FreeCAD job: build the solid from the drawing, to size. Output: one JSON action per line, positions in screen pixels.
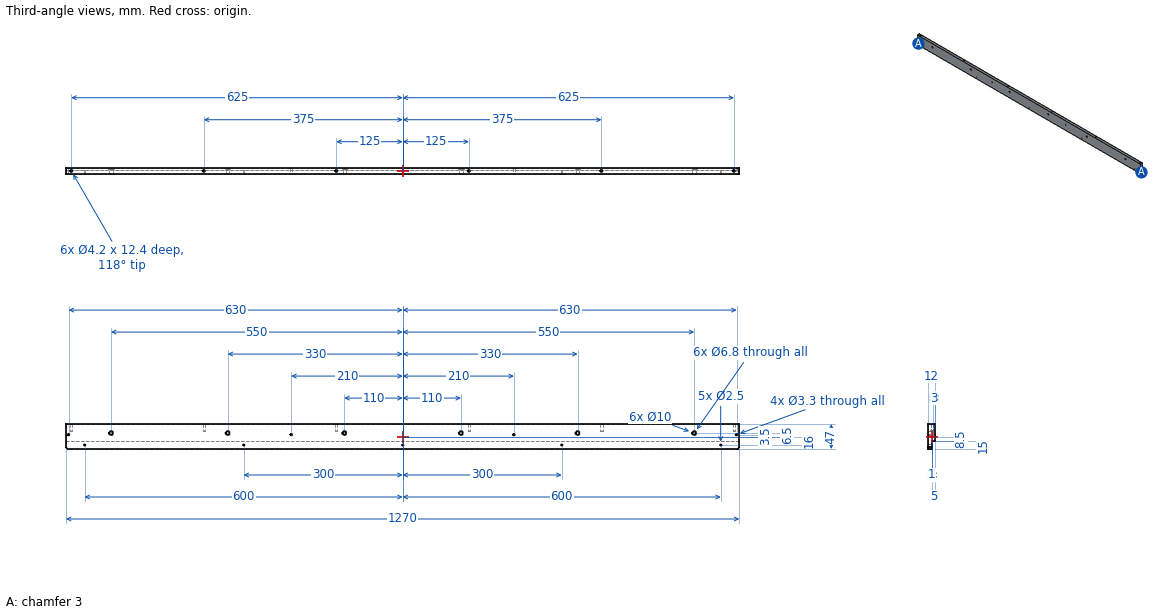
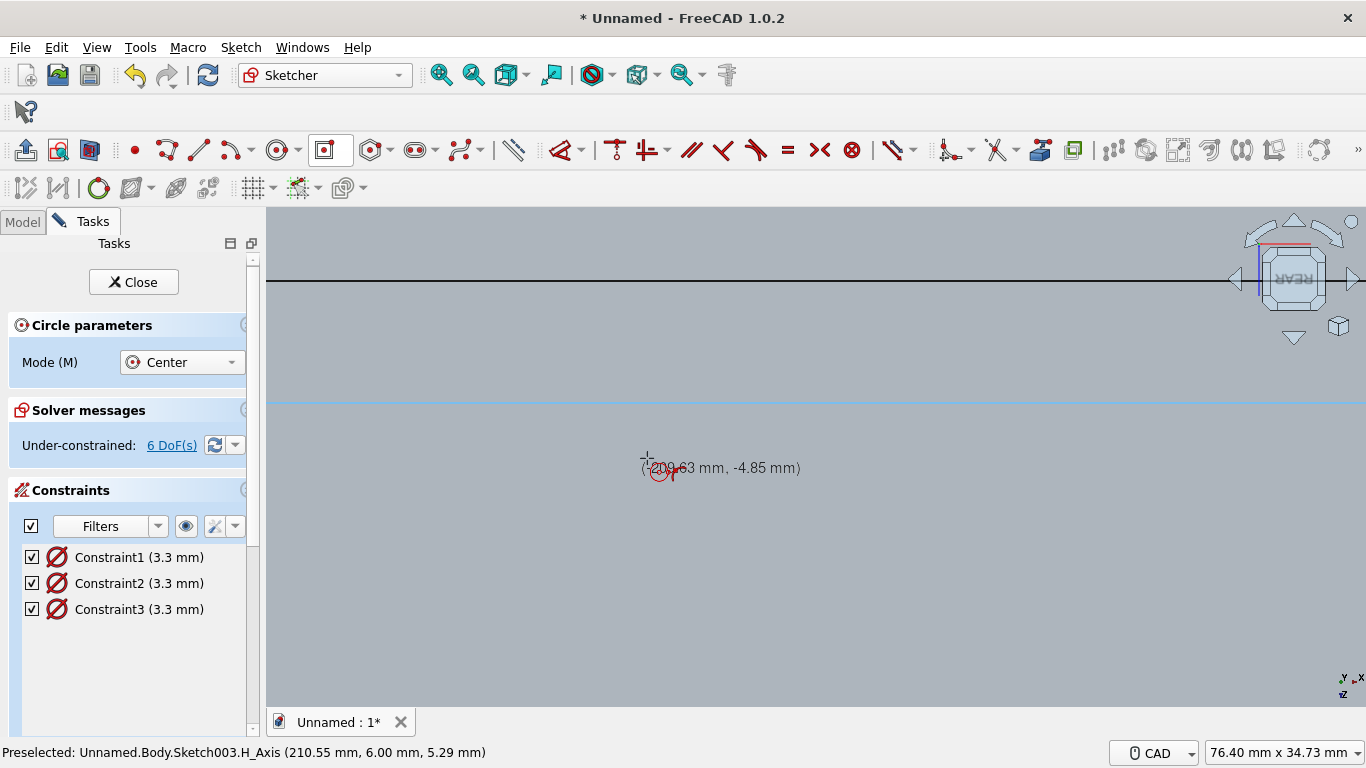
{"action": "scroll", "coordinate": [624, 458], "scroll_direction": "down", "scroll_amount": 16}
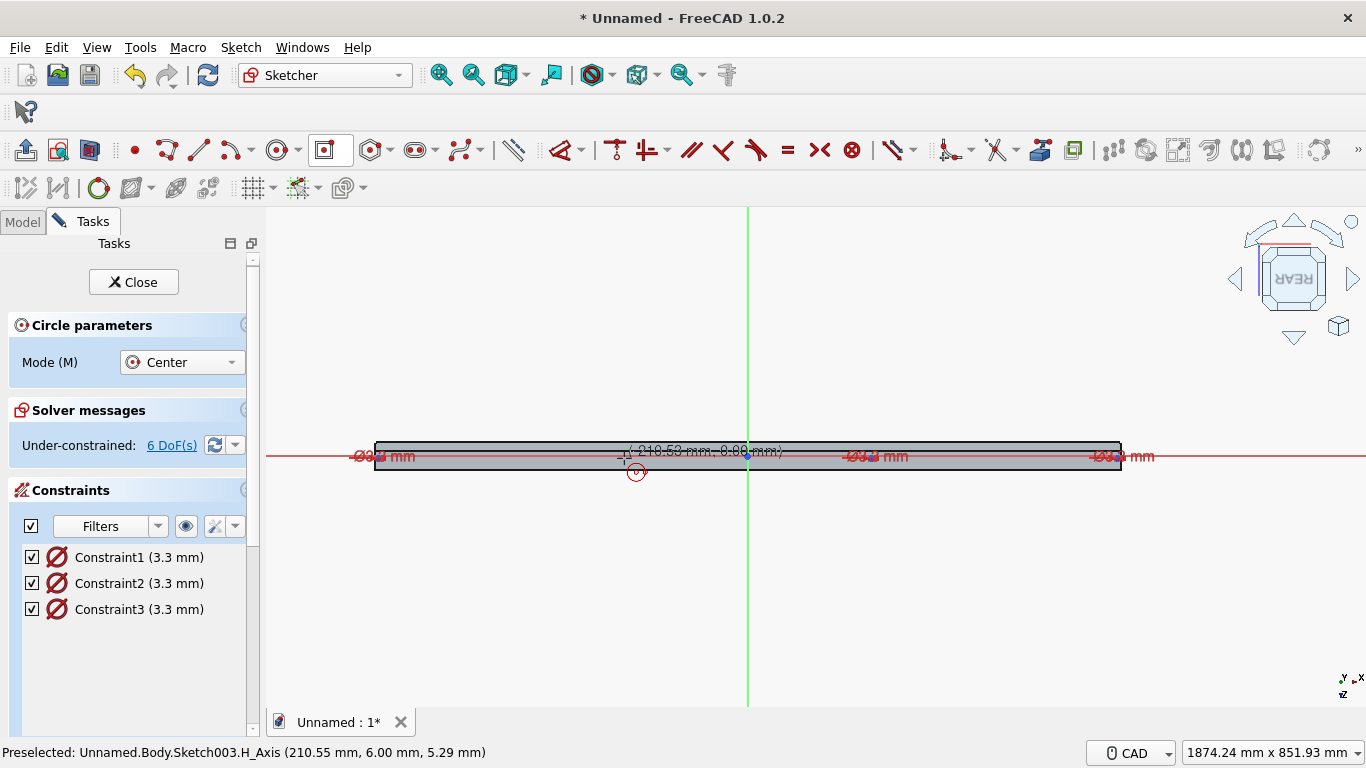
{"action": "scroll", "coordinate": [625, 458], "scroll_direction": "up", "scroll_amount": 11}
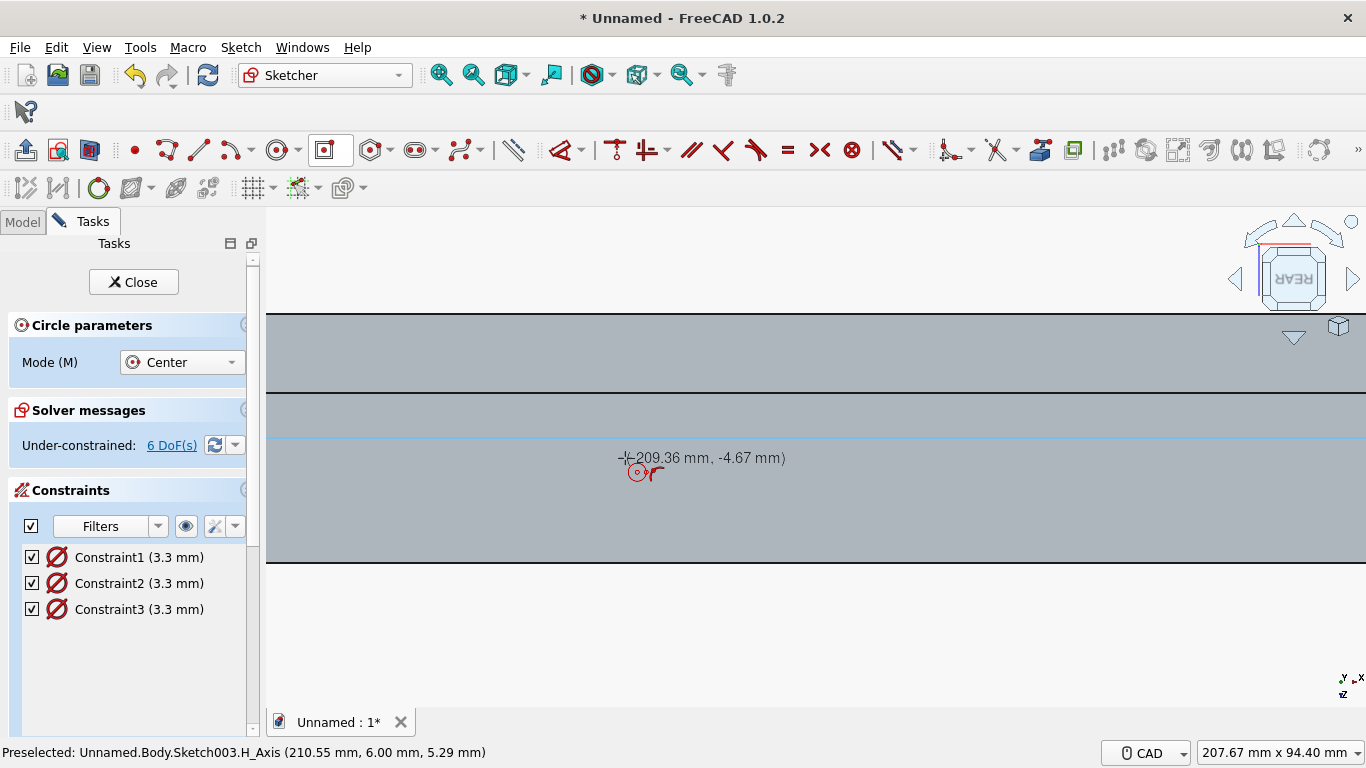
{"action": "left_click", "coordinate": [619, 457]}
{"action": "mouse_move", "coordinate": [625, 463]}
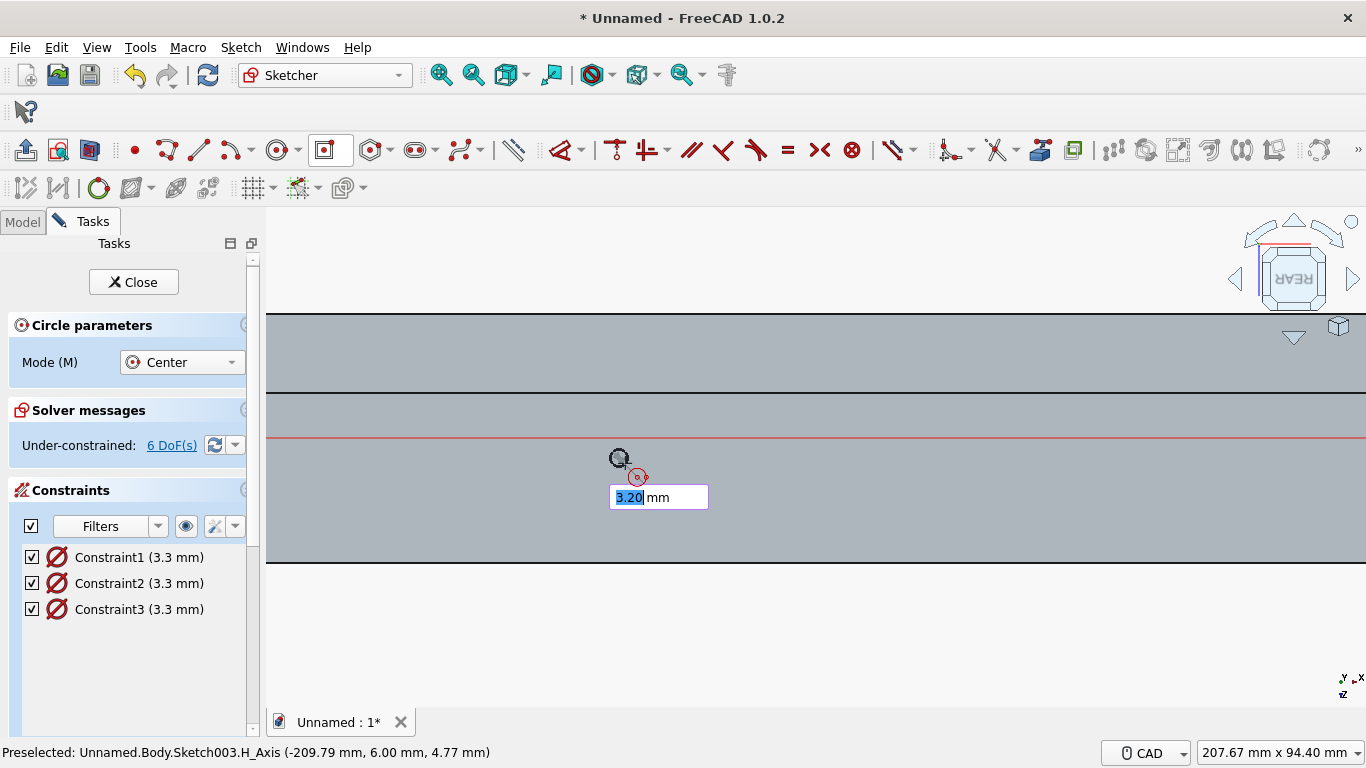
{"action": "type", "text": "3.3"}
{"action": "key", "text": "Return"}
{"action": "key", "text": "Escape"}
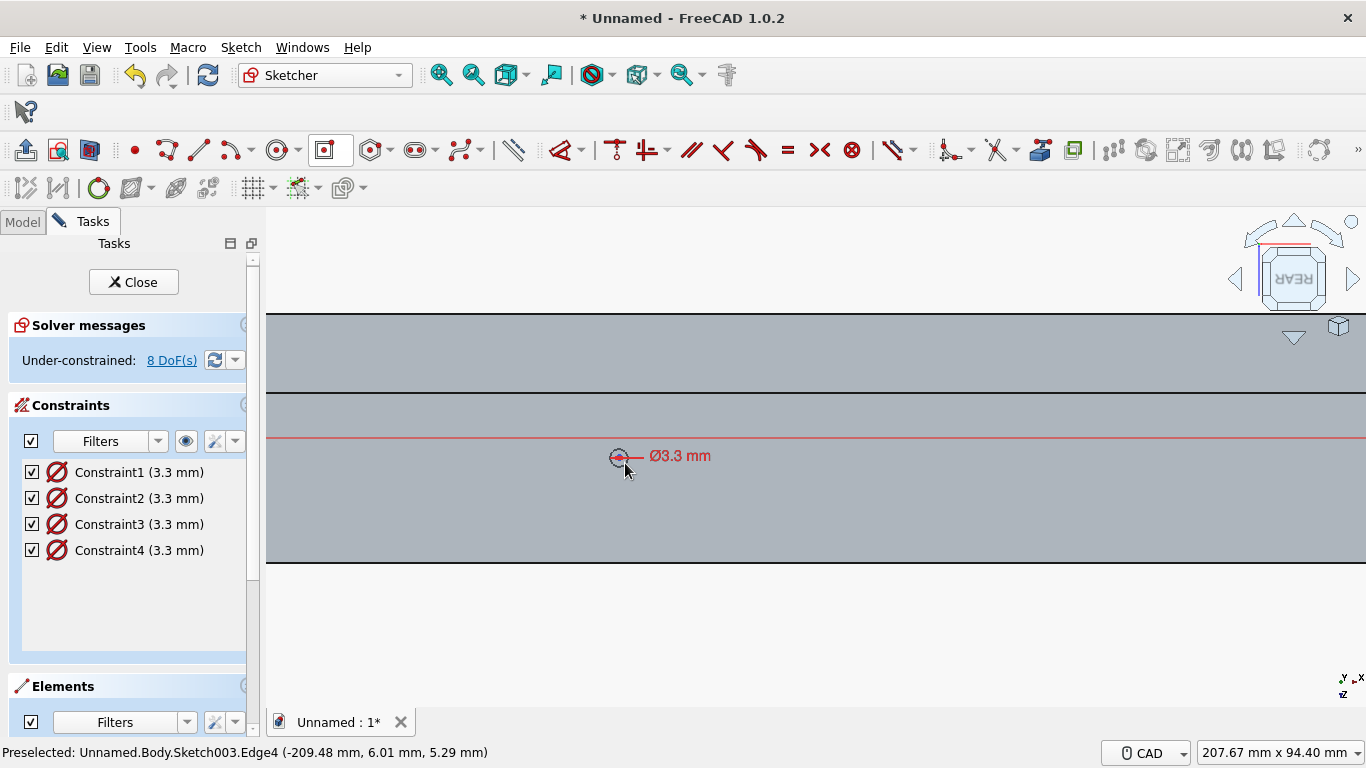
{"action": "scroll", "coordinate": [649, 458], "scroll_direction": "down", "scroll_amount": 12}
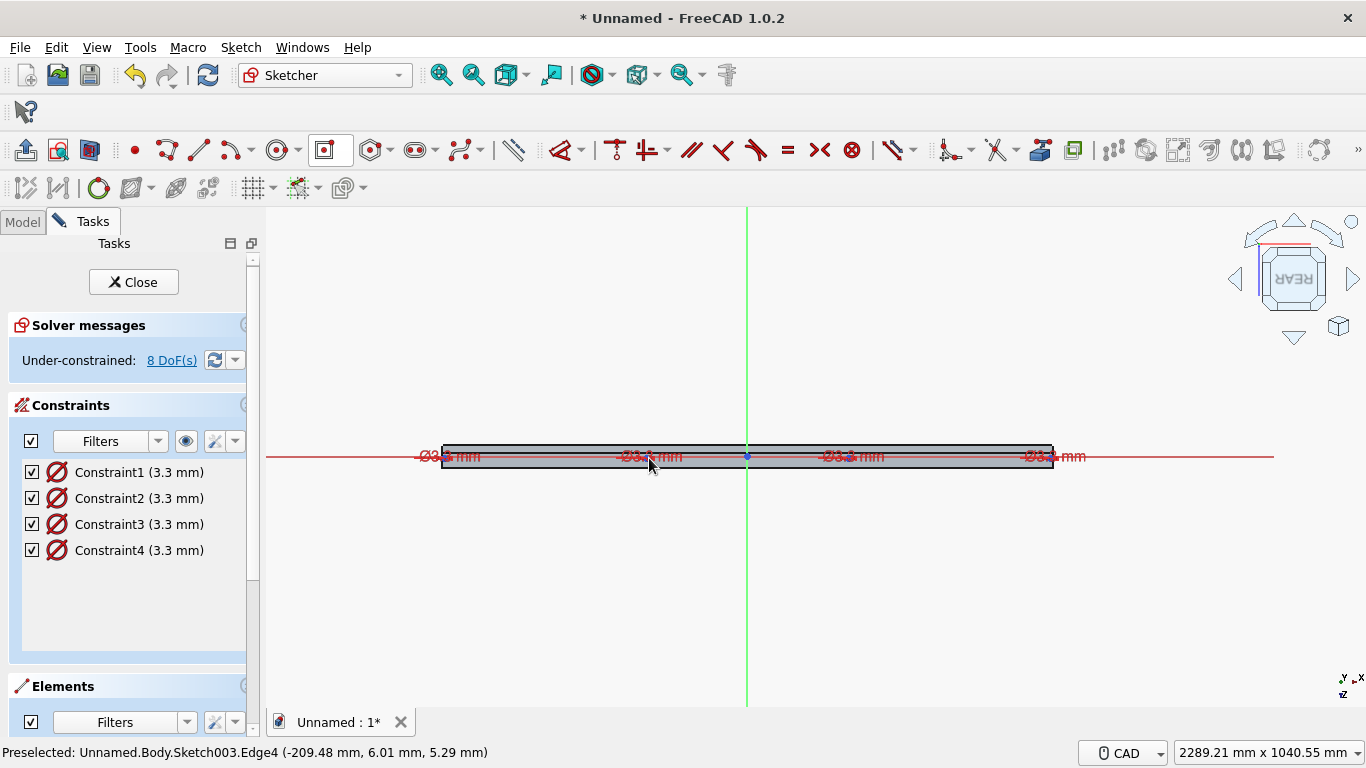
{"action": "left_click", "coordinate": [1050, 458]}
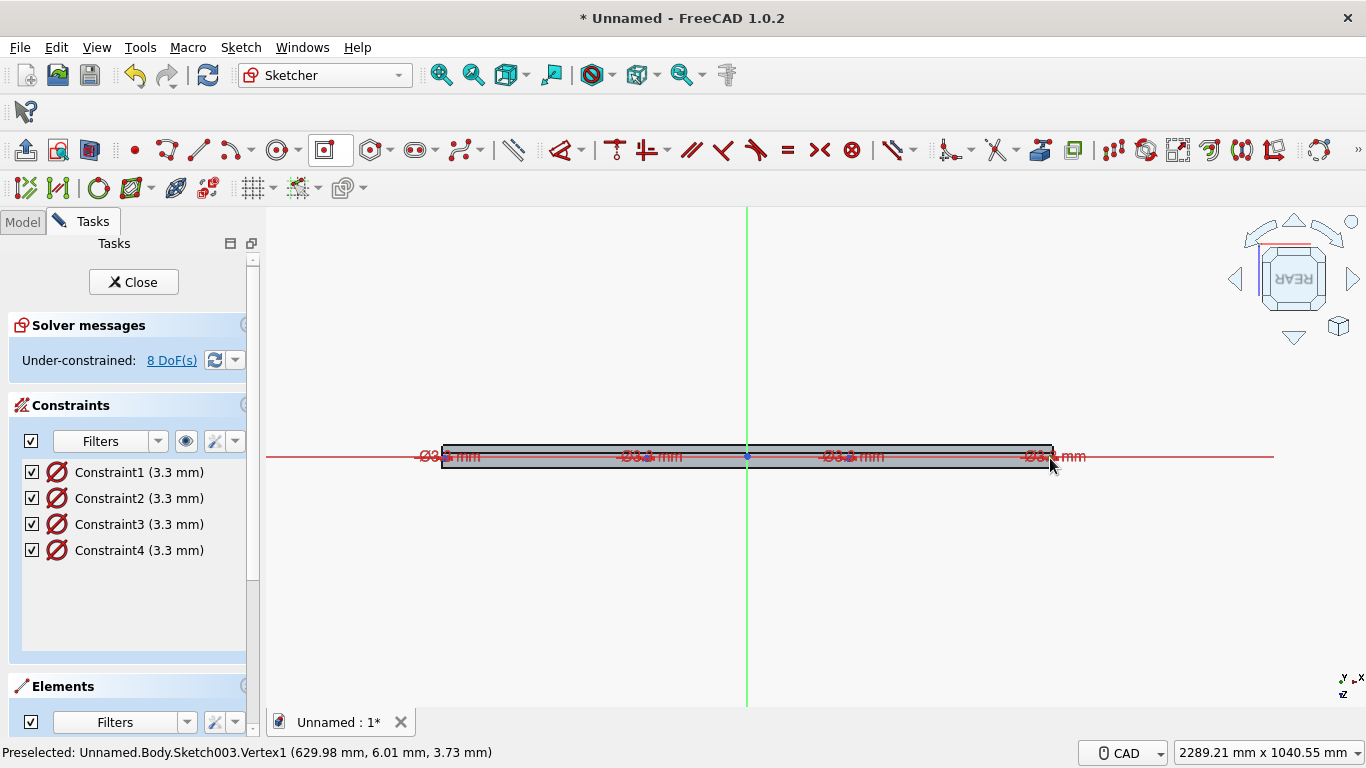
{"action": "left_click", "coordinate": [445, 458]}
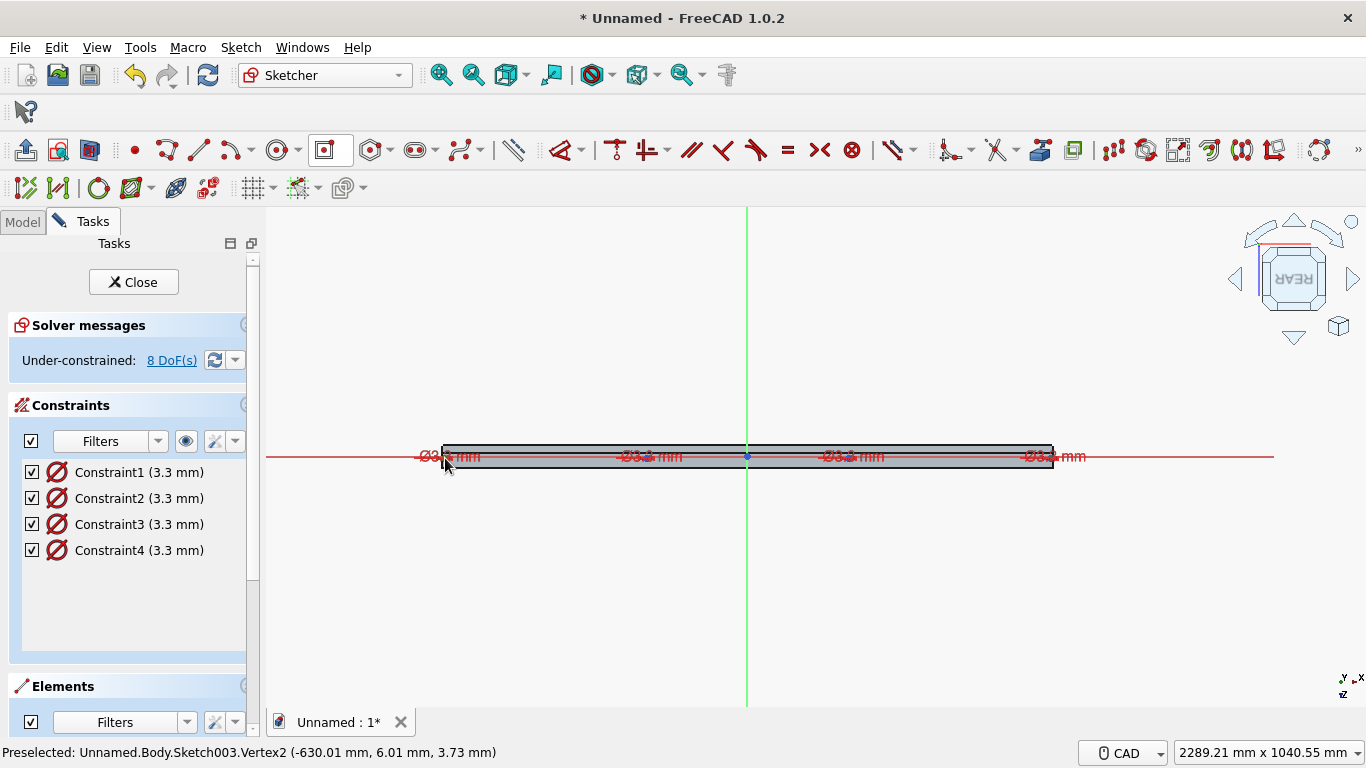
{"action": "left_click", "coordinate": [670, 150]}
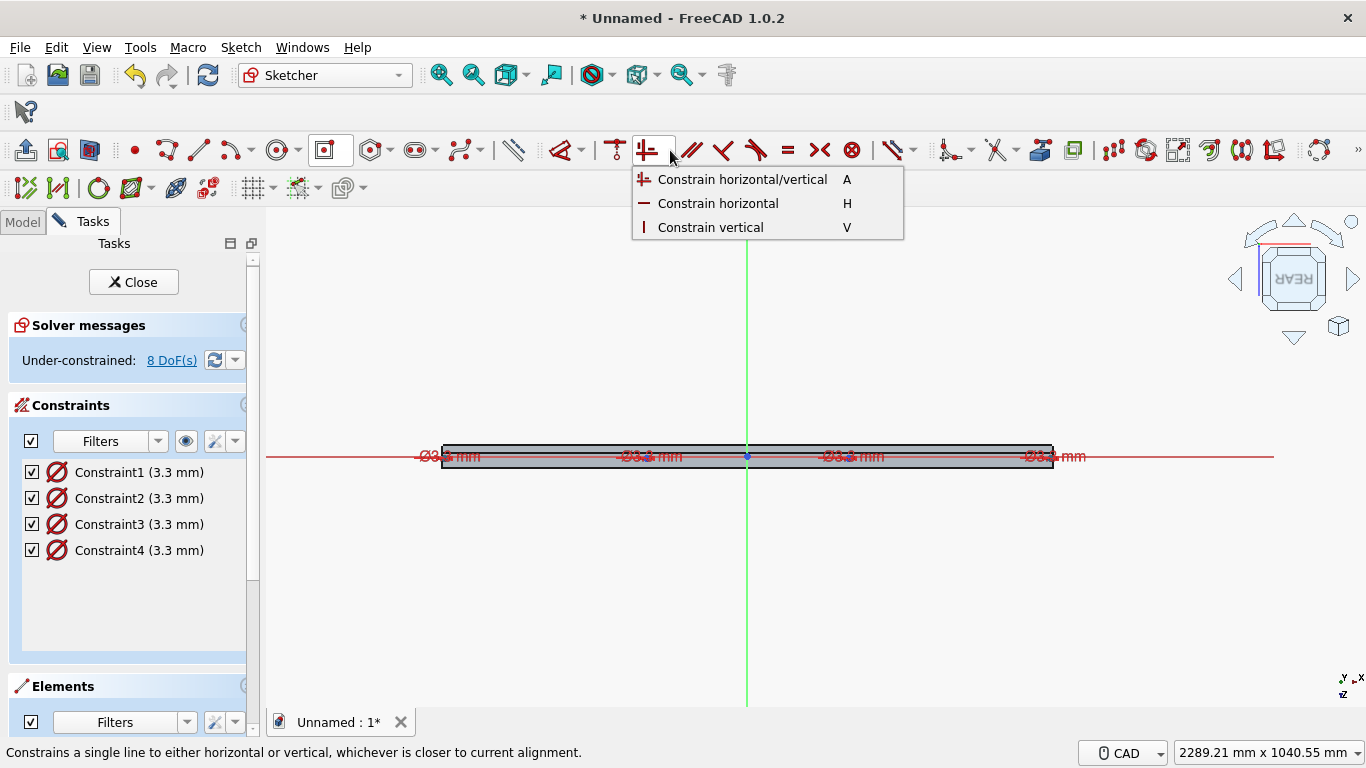
{"action": "left_click", "coordinate": [768, 203]}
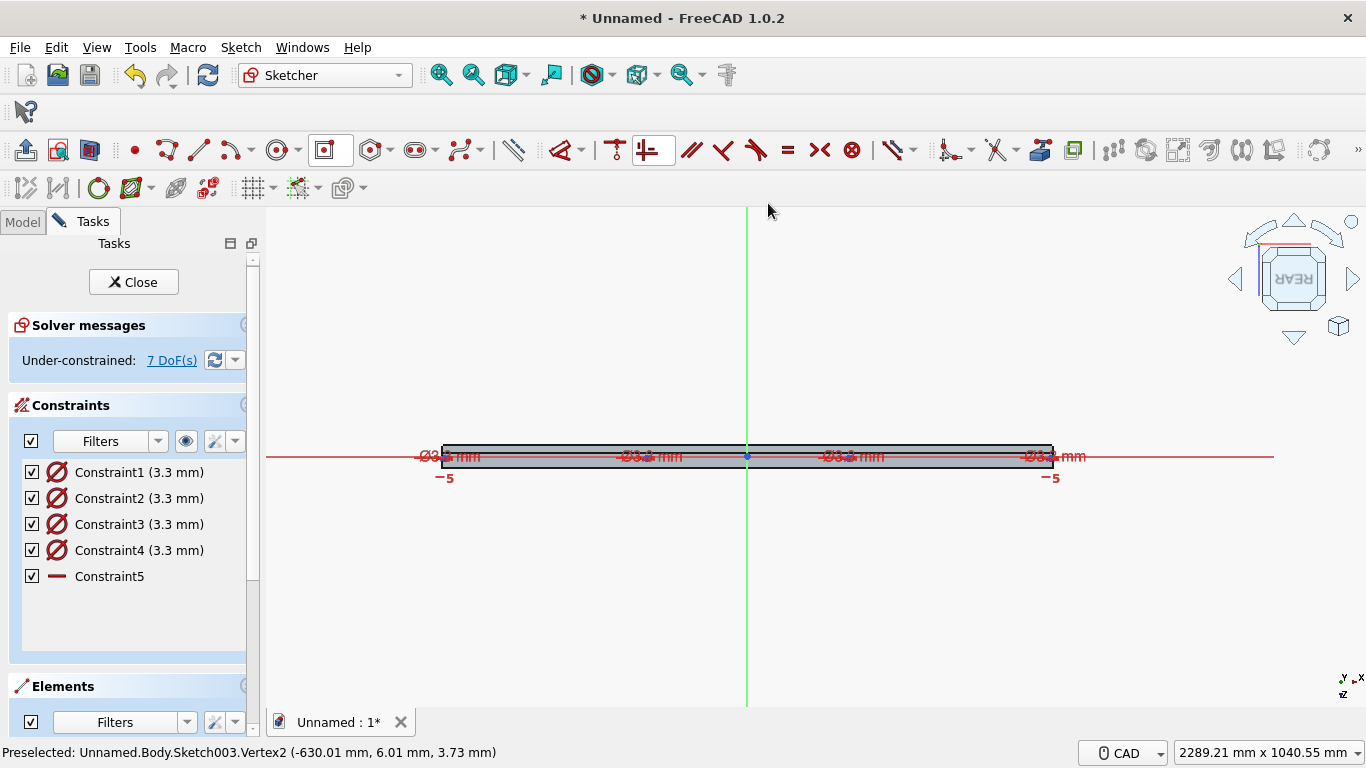
{"action": "left_click", "coordinate": [1050, 458]}